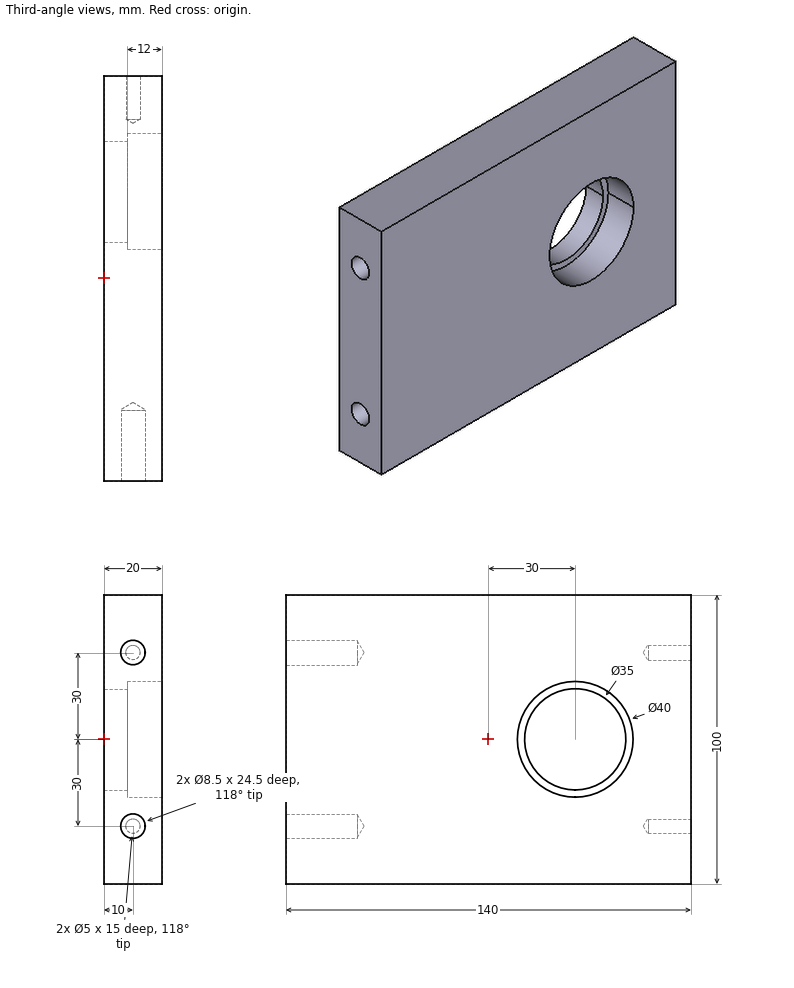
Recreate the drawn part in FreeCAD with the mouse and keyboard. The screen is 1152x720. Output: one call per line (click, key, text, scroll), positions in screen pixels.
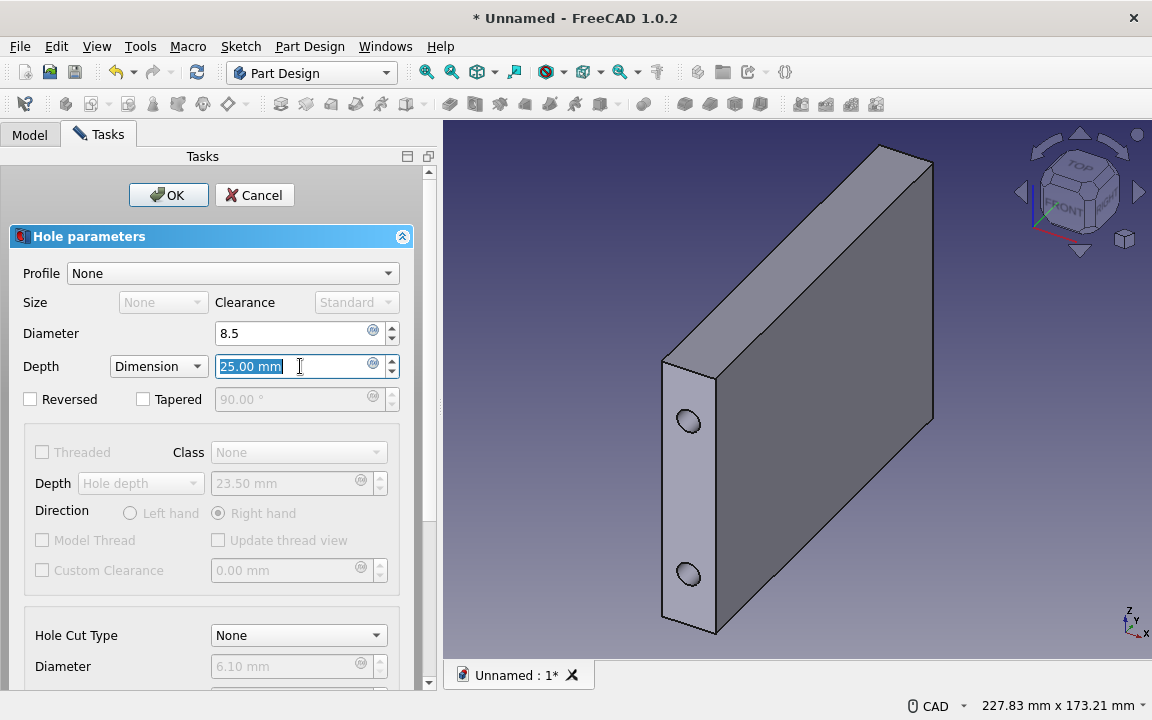
text(24.5)
key(Tab)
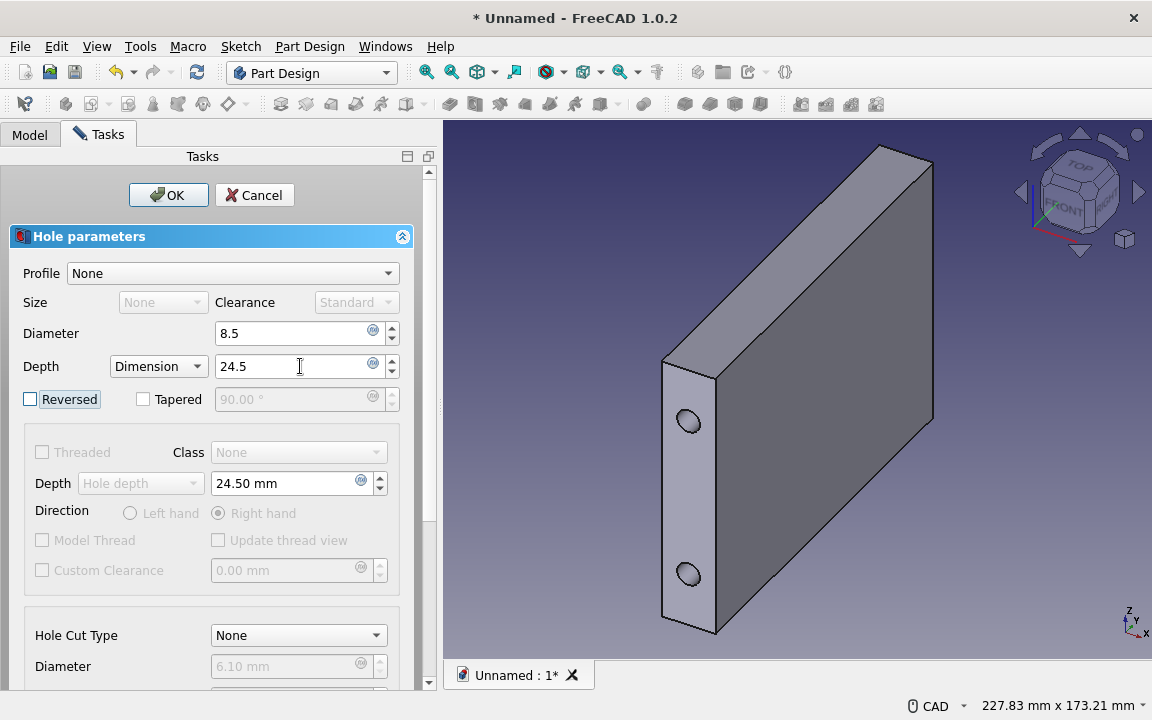
click(169, 195)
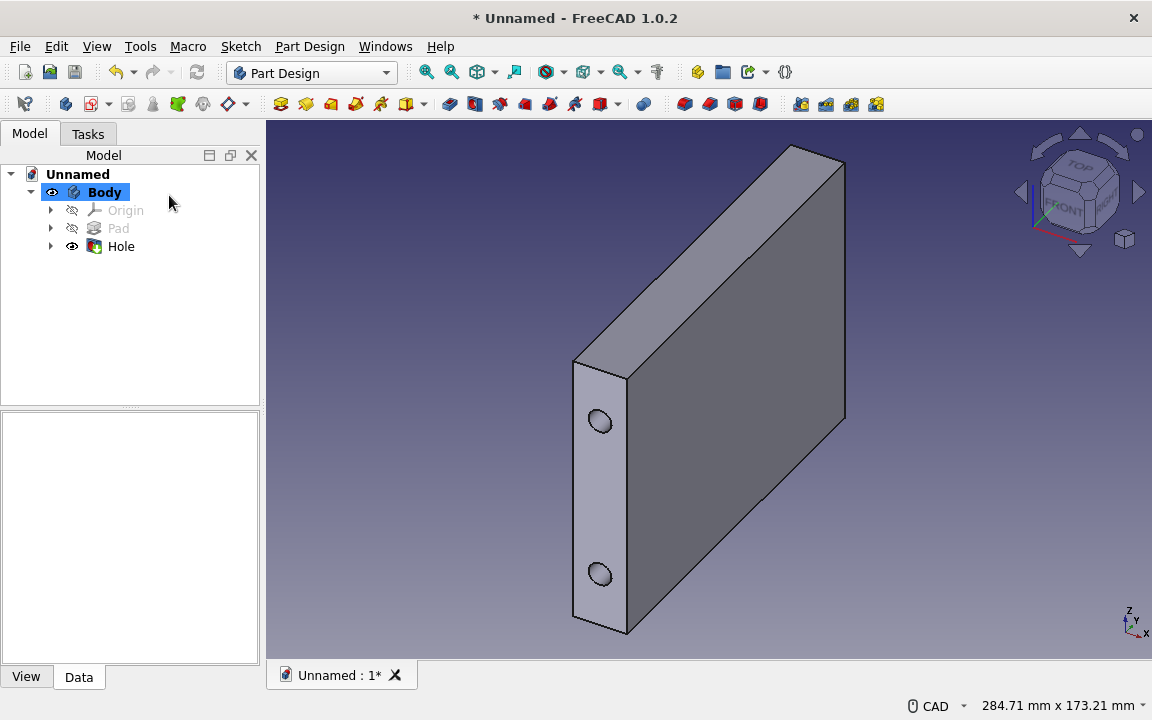
click(736, 397)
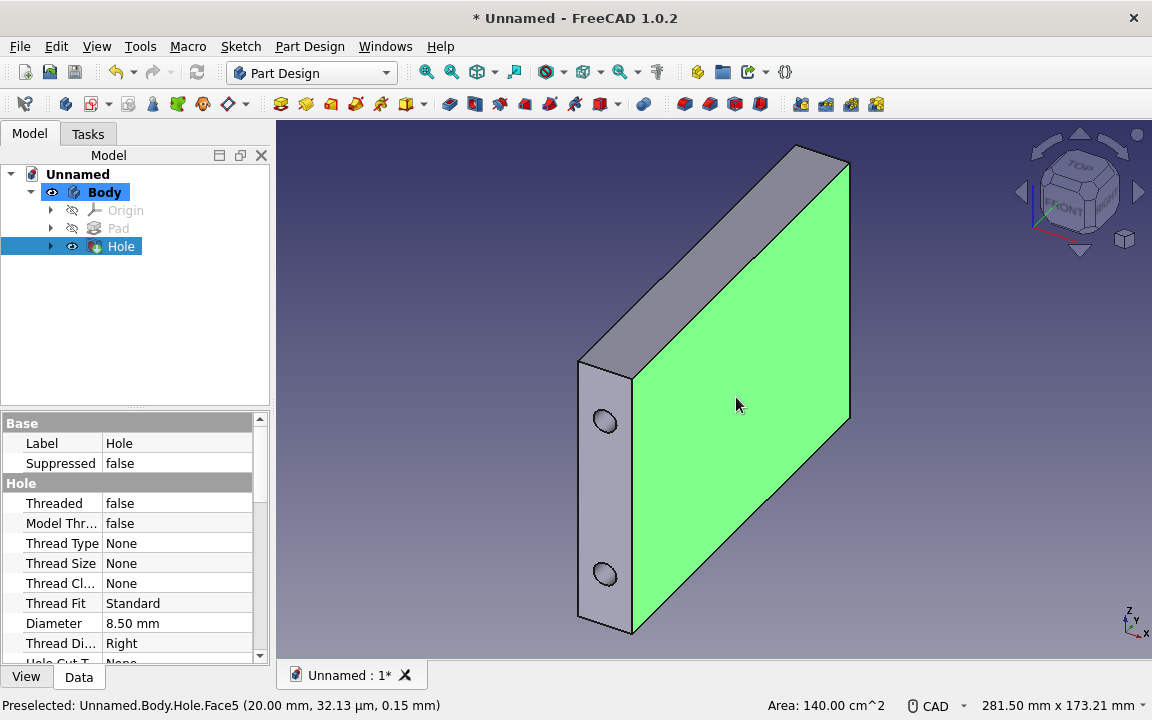
click(90, 104)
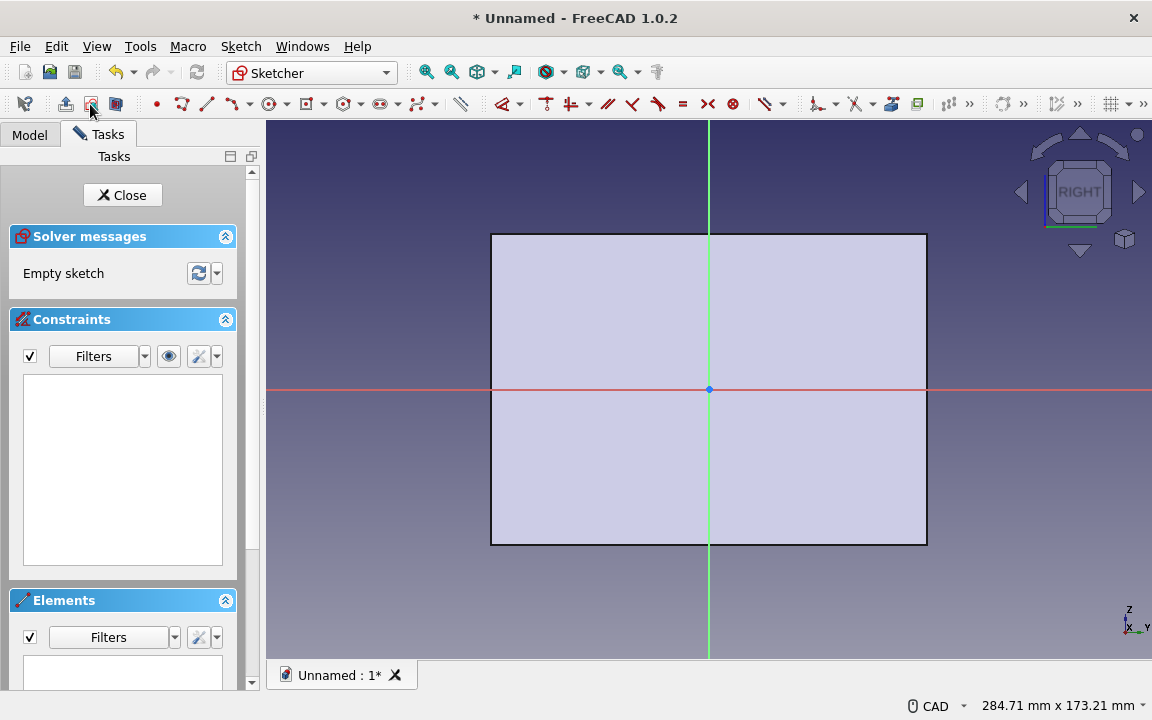
scroll(872, 390, up, 5)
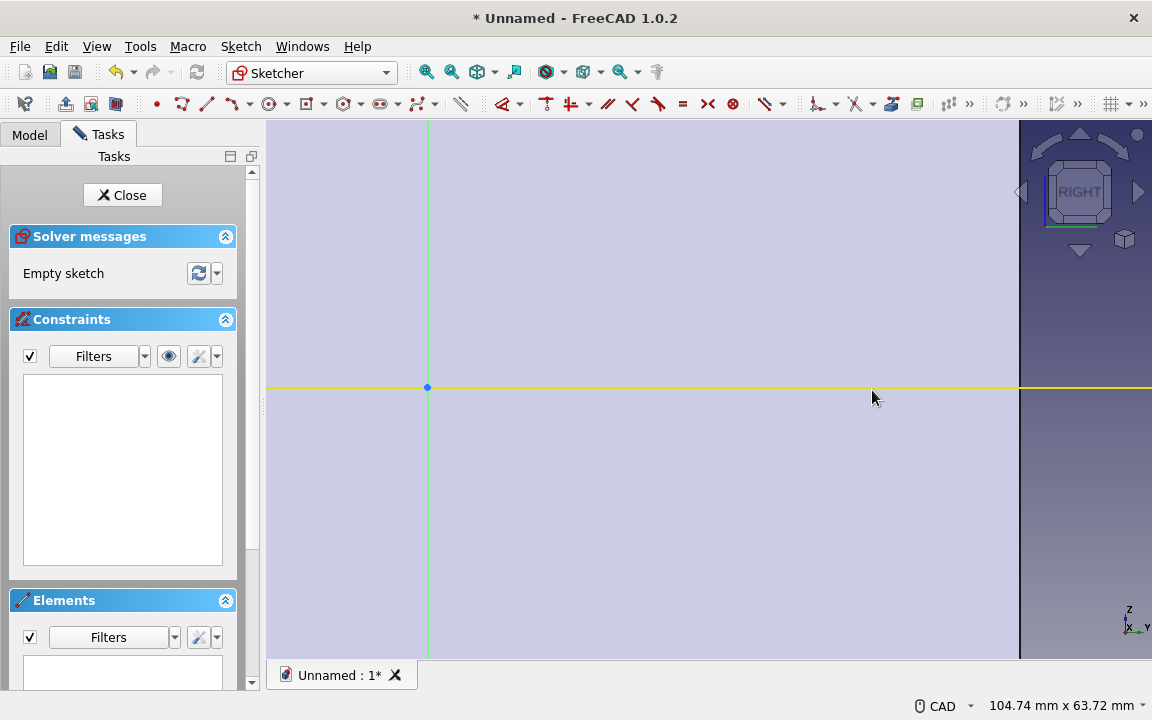
key(g)
key(c)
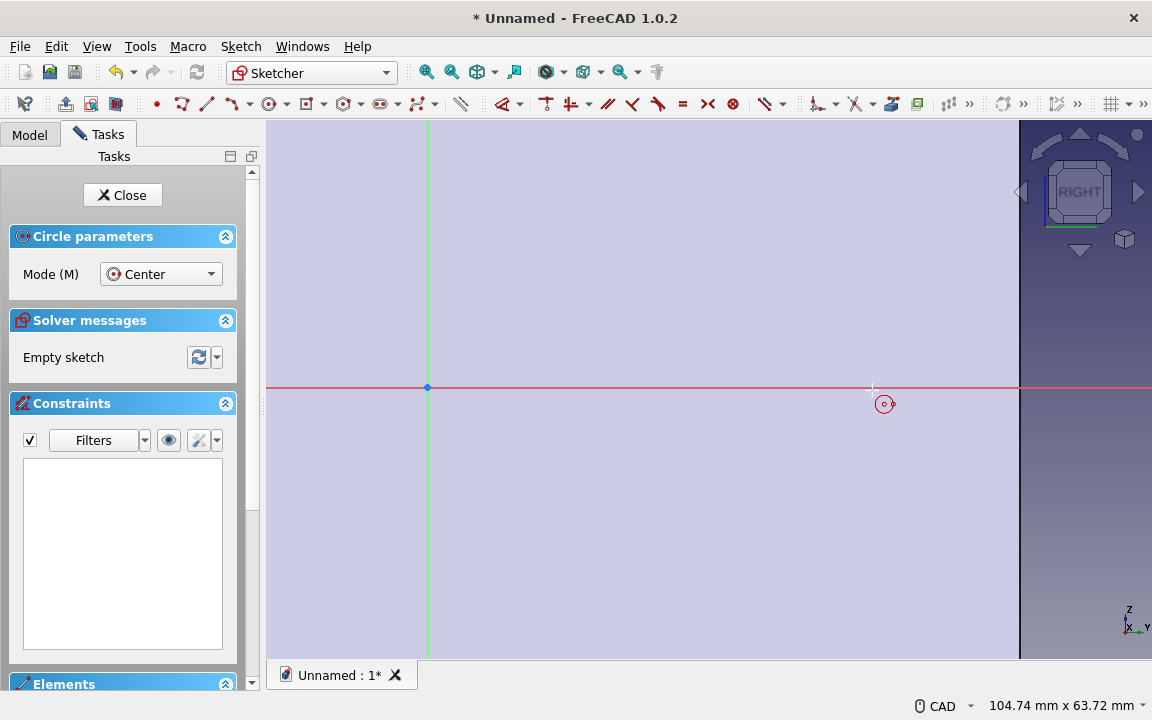
click(682, 388)
move(801, 268)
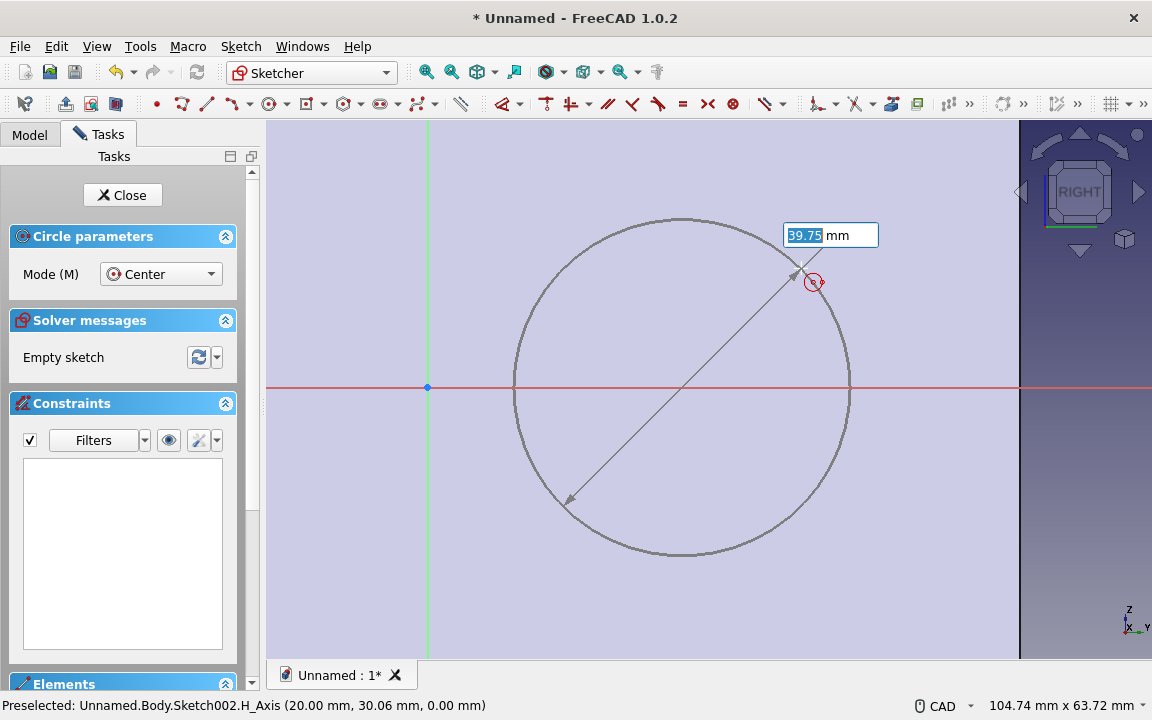
text(40)
key(Return)
key(Escape)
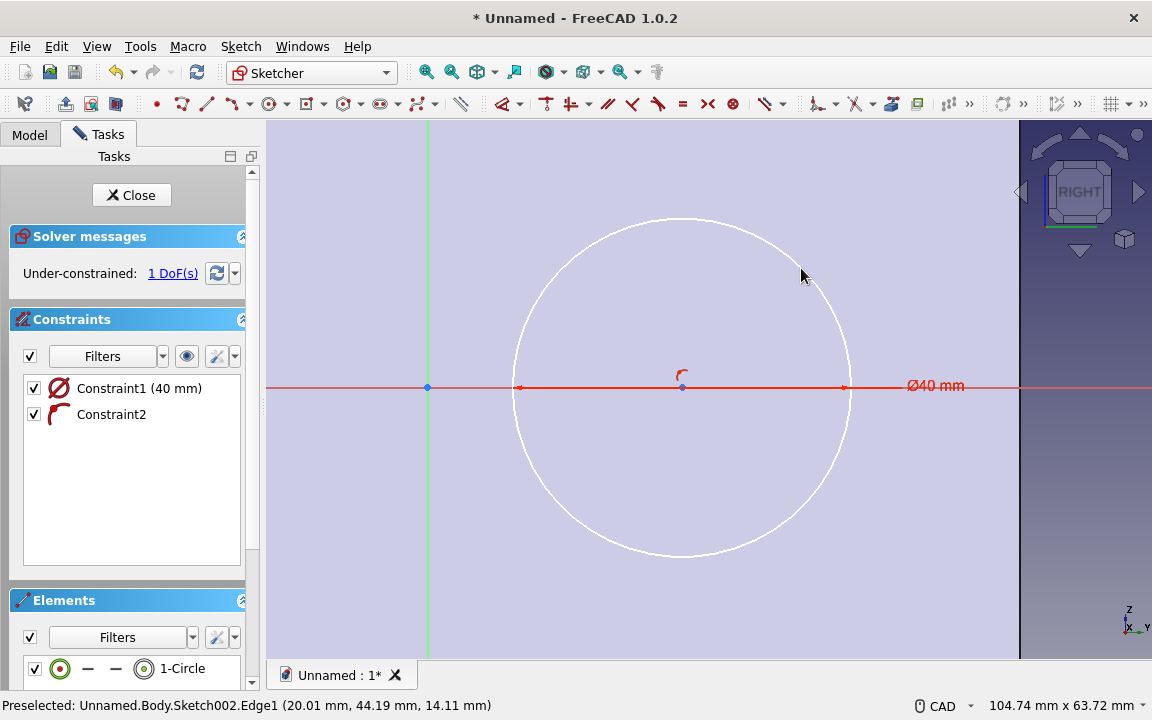
key(d)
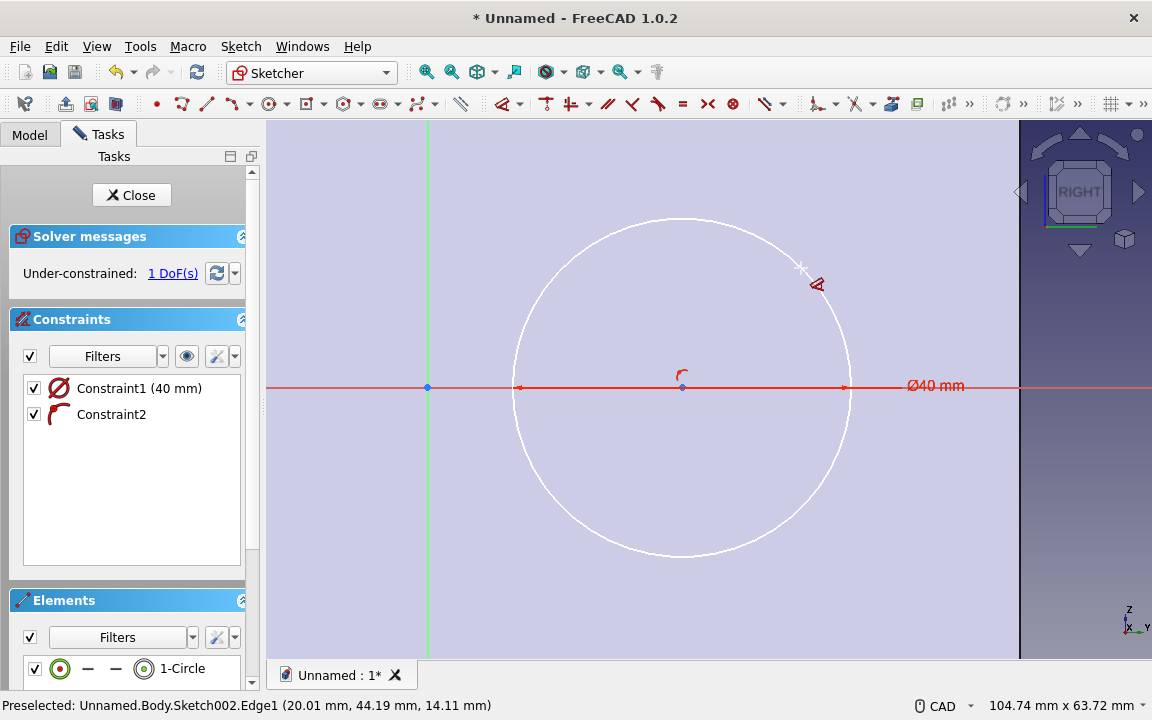
click(682, 388)
click(555, 422)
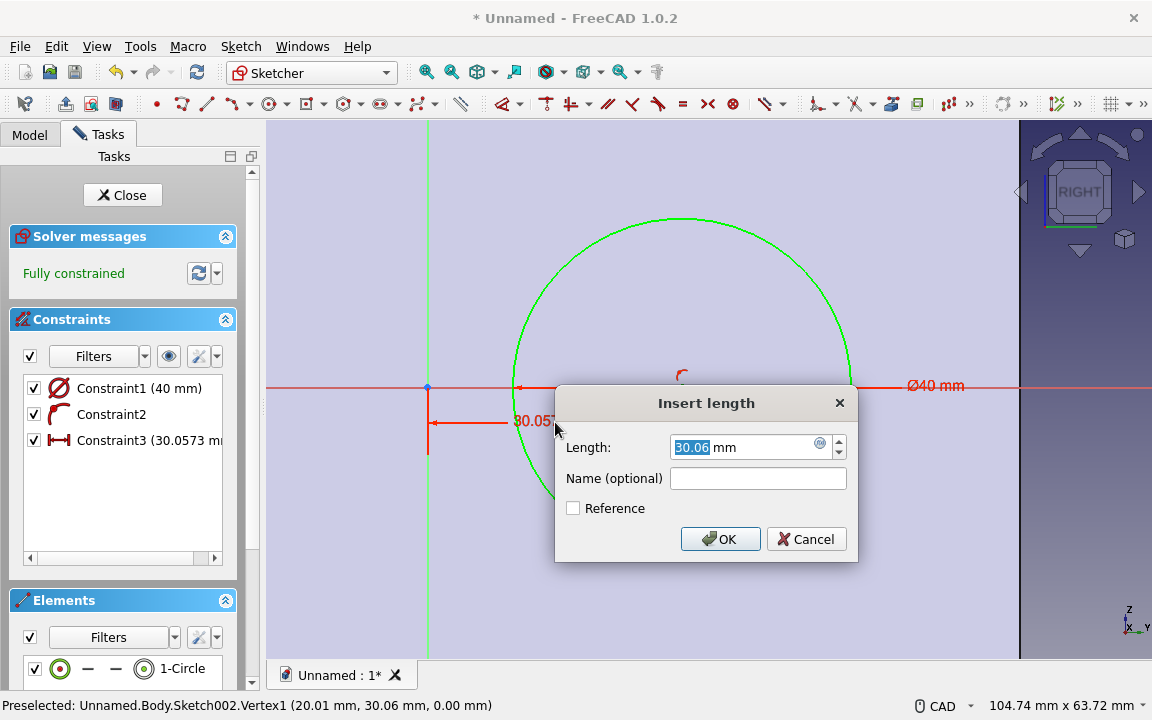
text(30)
key(Return)
key(Escape)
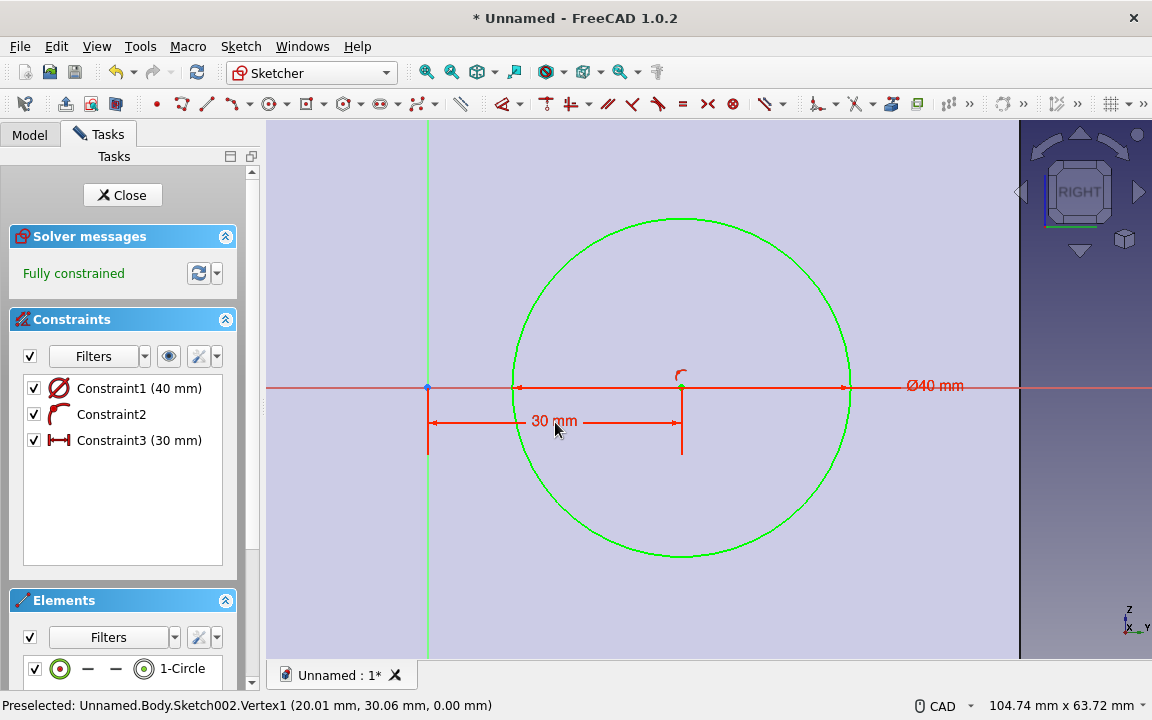
click(123, 195)